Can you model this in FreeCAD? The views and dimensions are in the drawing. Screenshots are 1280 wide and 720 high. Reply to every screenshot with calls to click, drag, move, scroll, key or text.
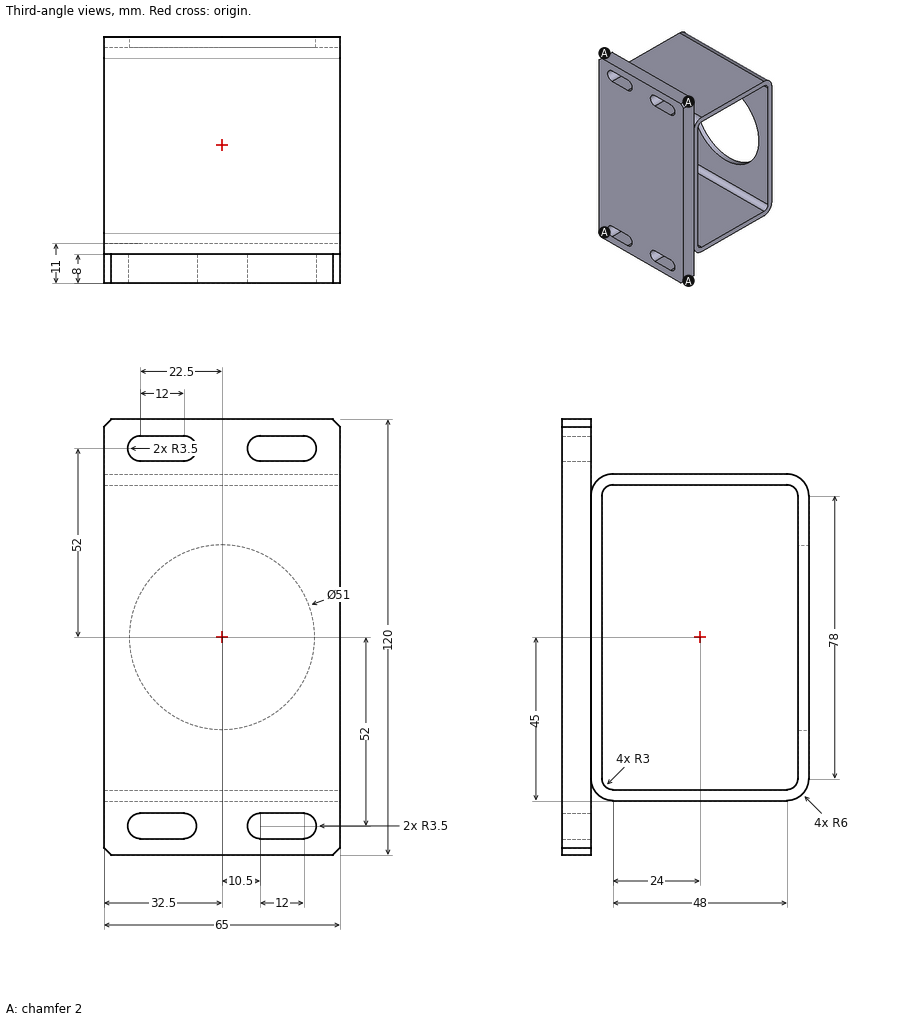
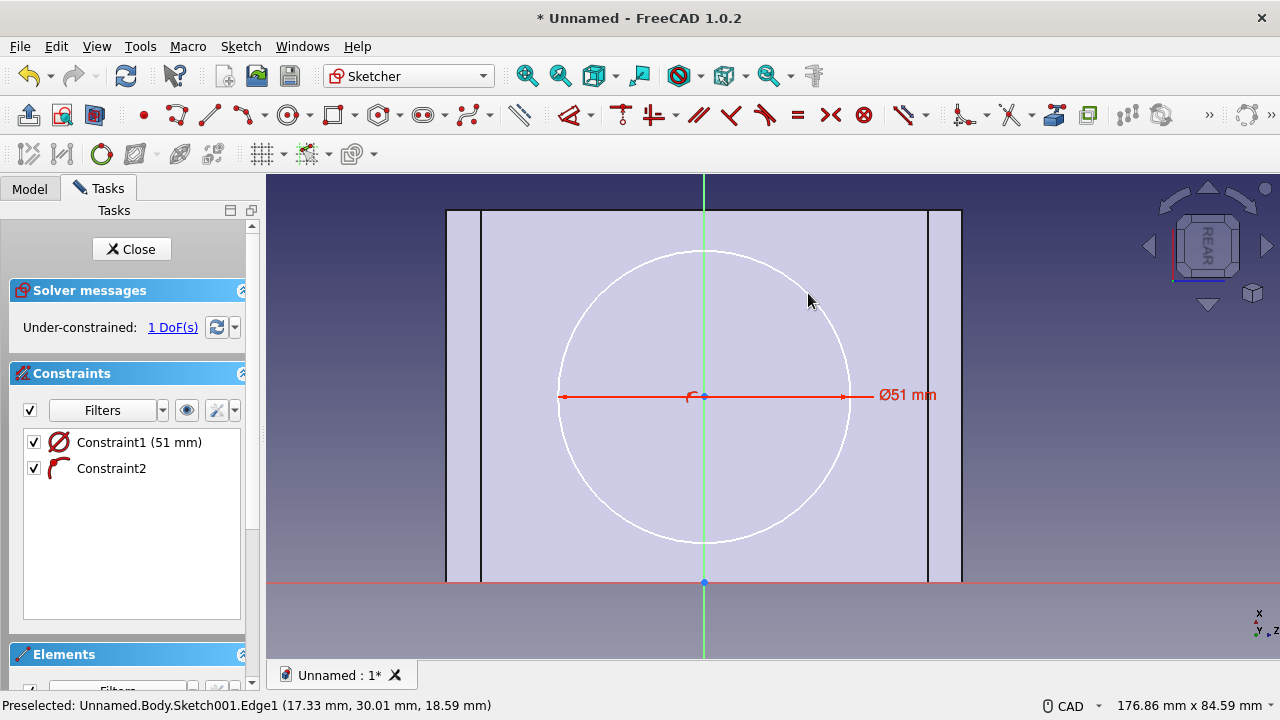
click(568, 116)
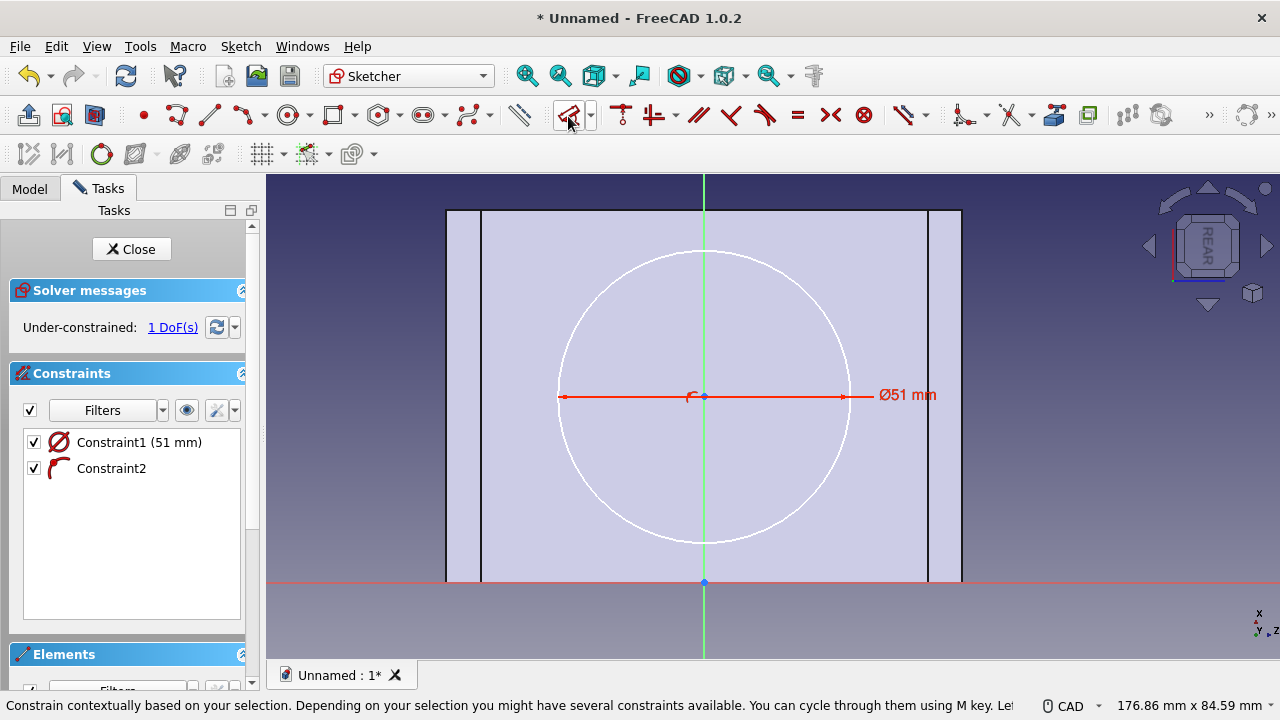
click(704, 397)
click(738, 490)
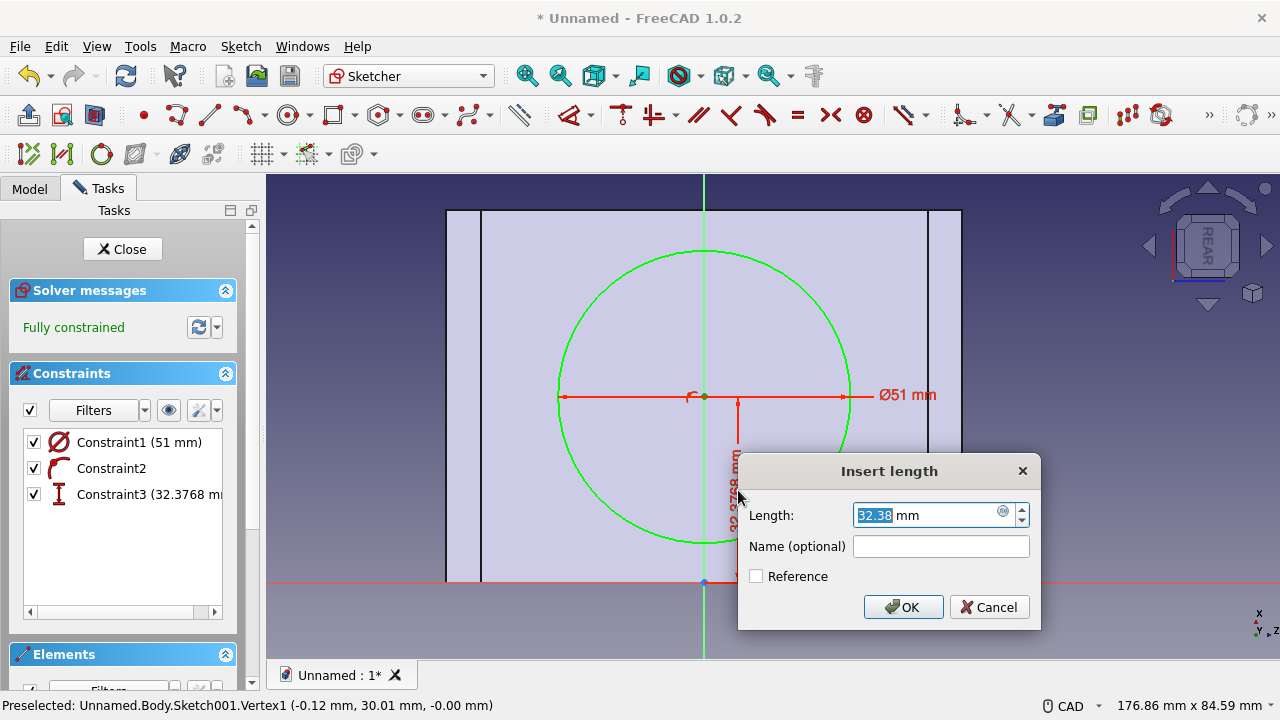
text(32.5)
key(Return)
key(Escape)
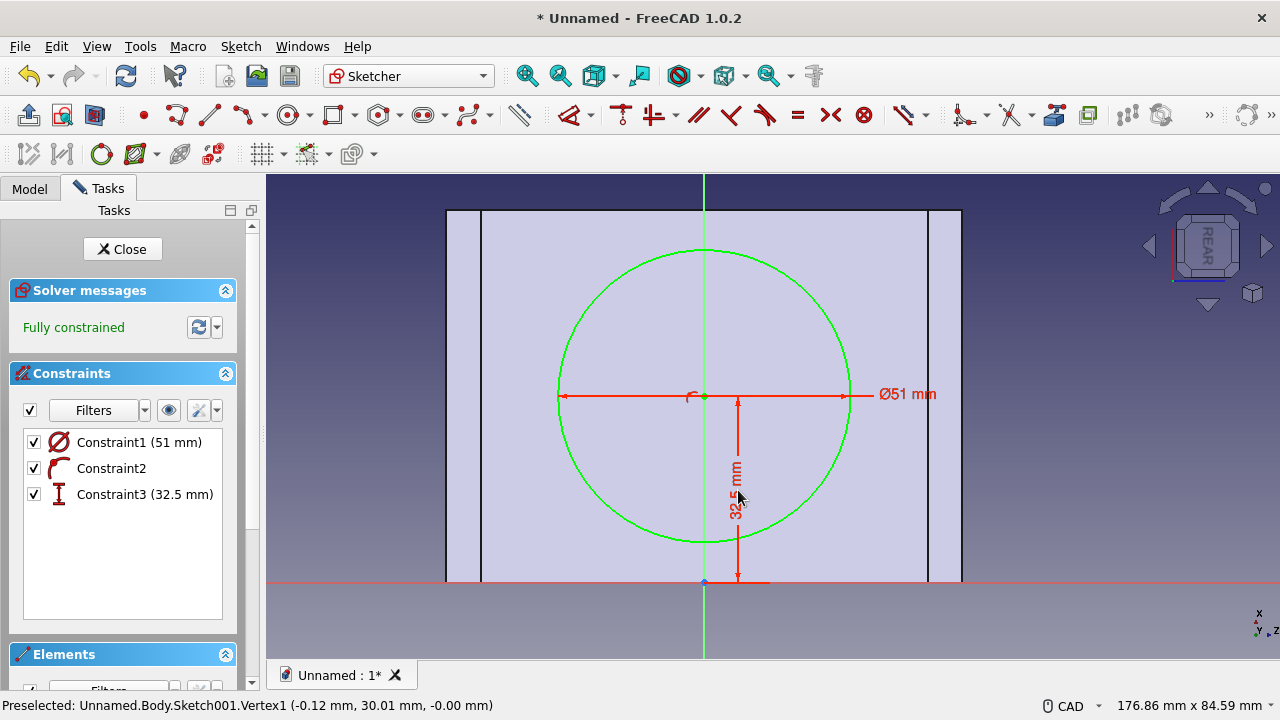
click(123, 249)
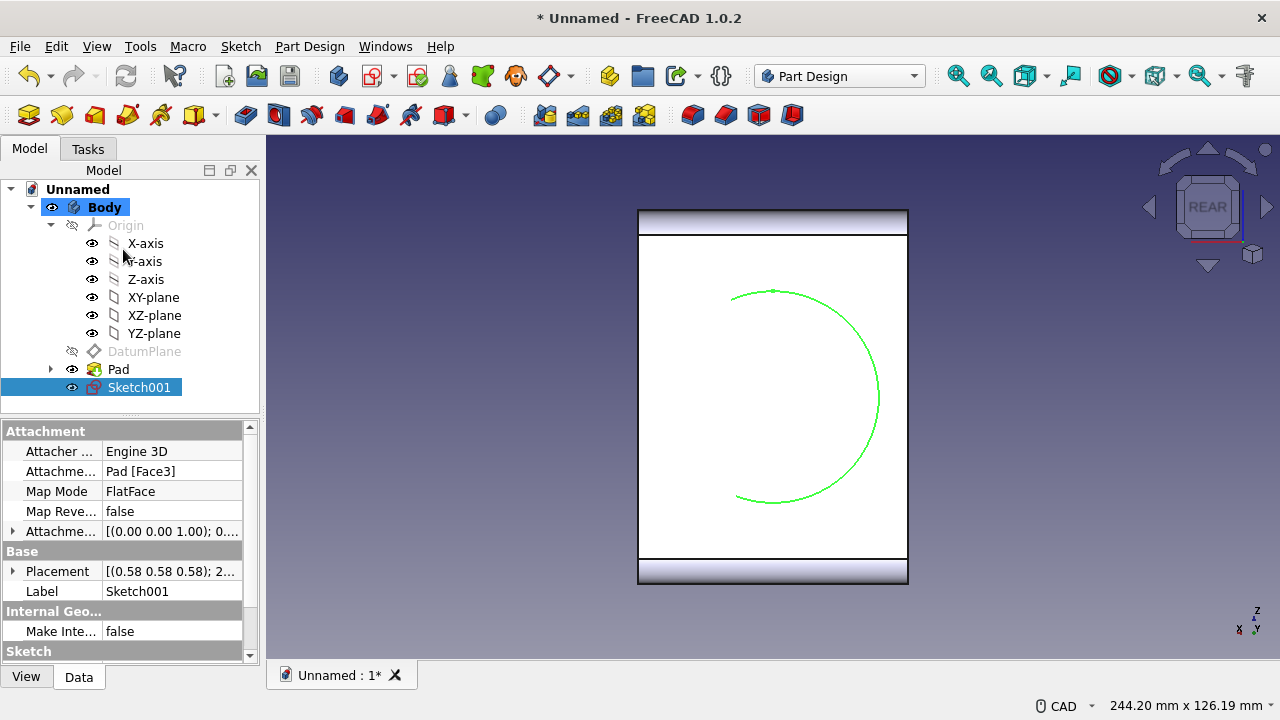
click(246, 116)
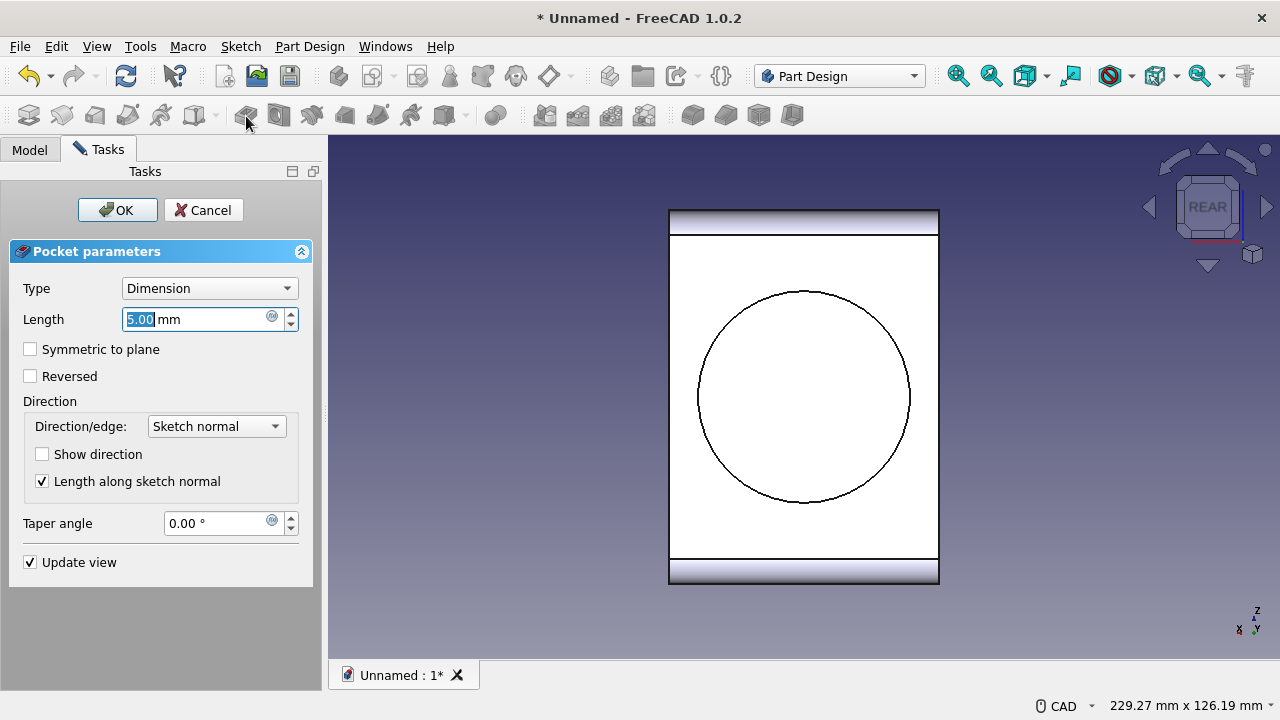
click(210, 288)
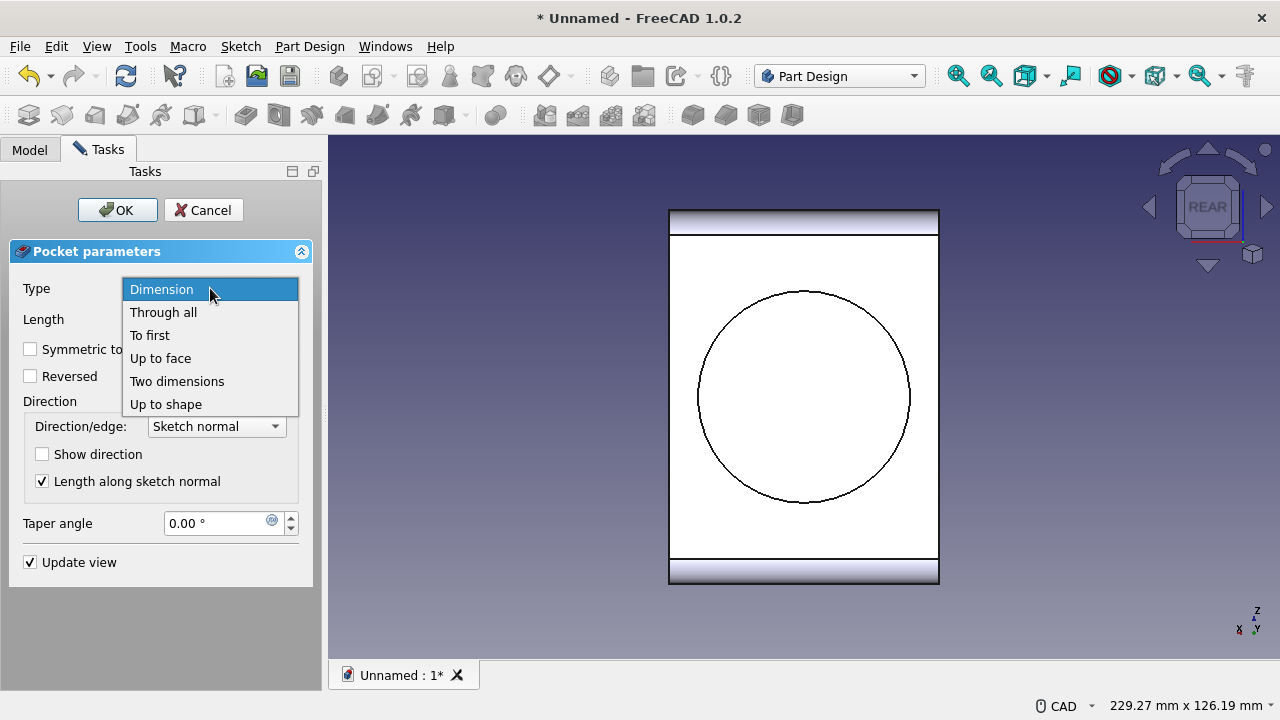
click(208, 336)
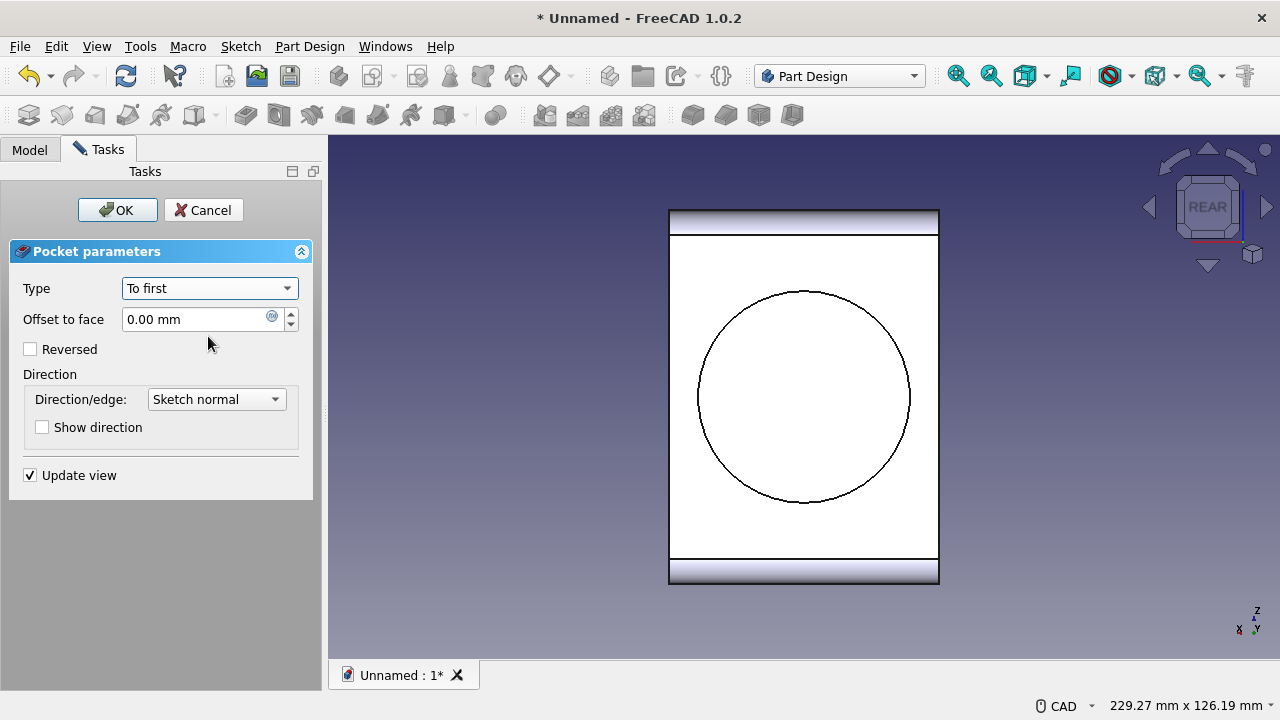
click(118, 210)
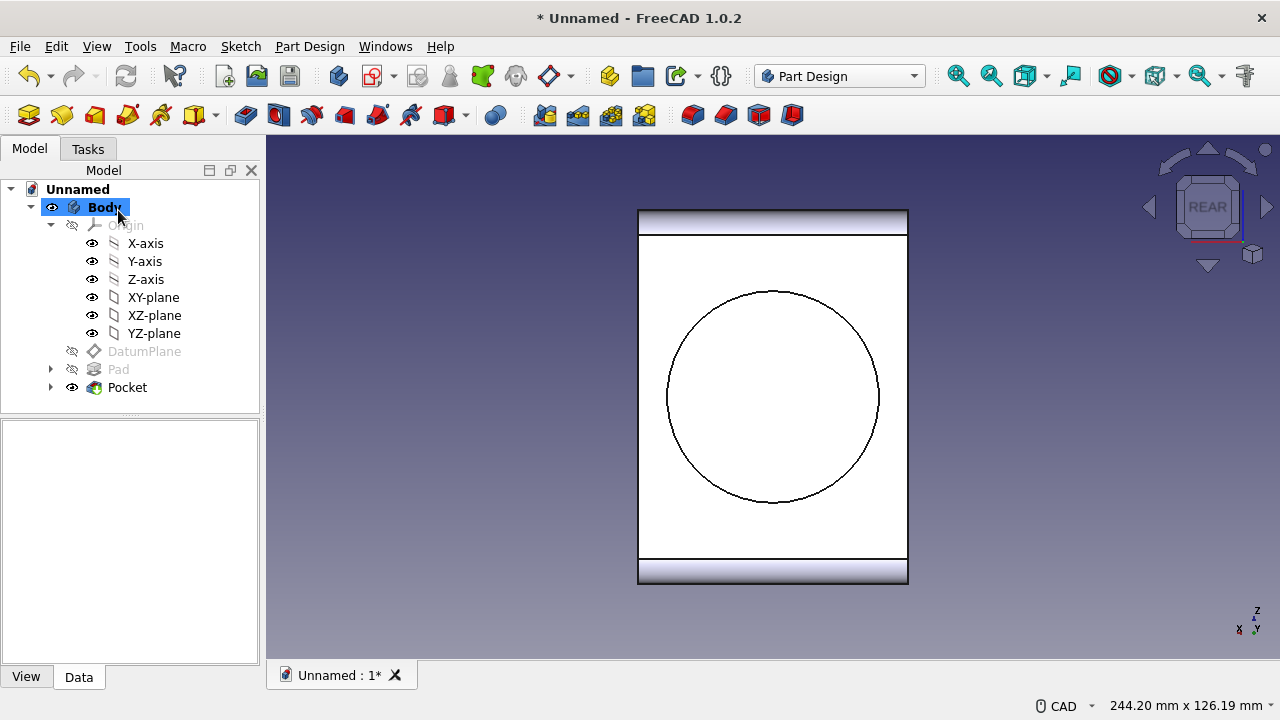
click(339, 76)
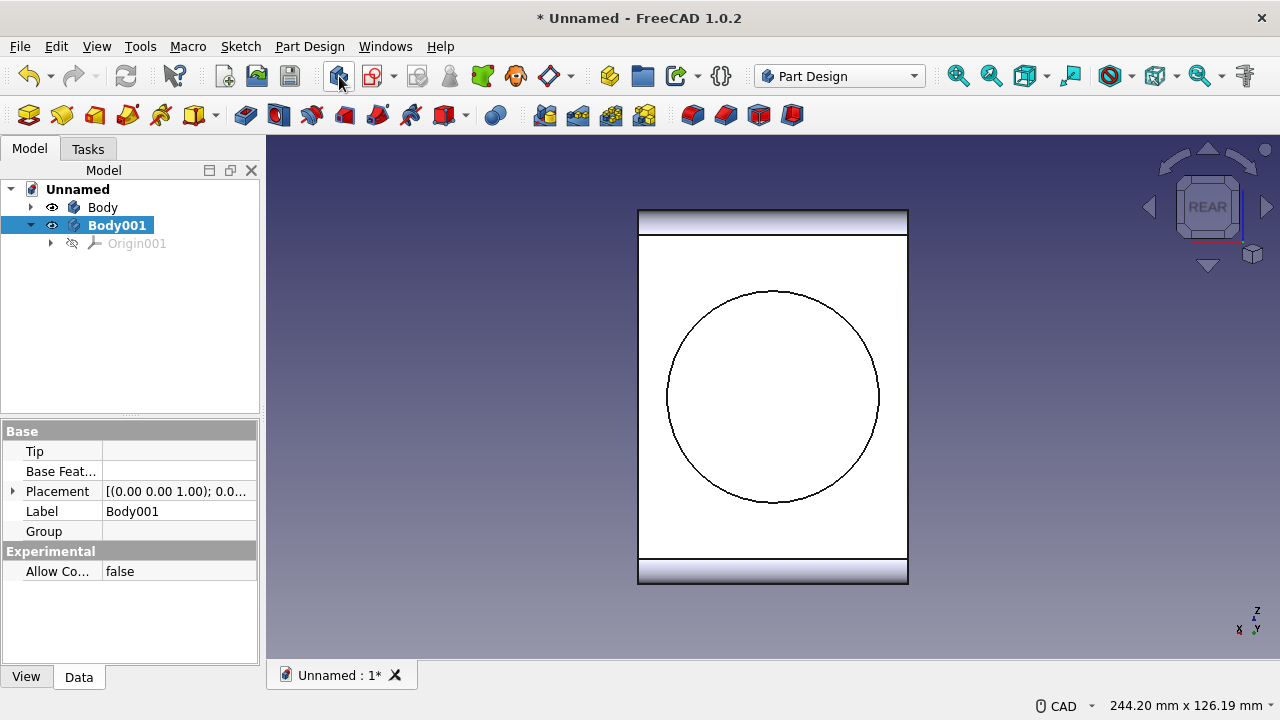
click(51, 243)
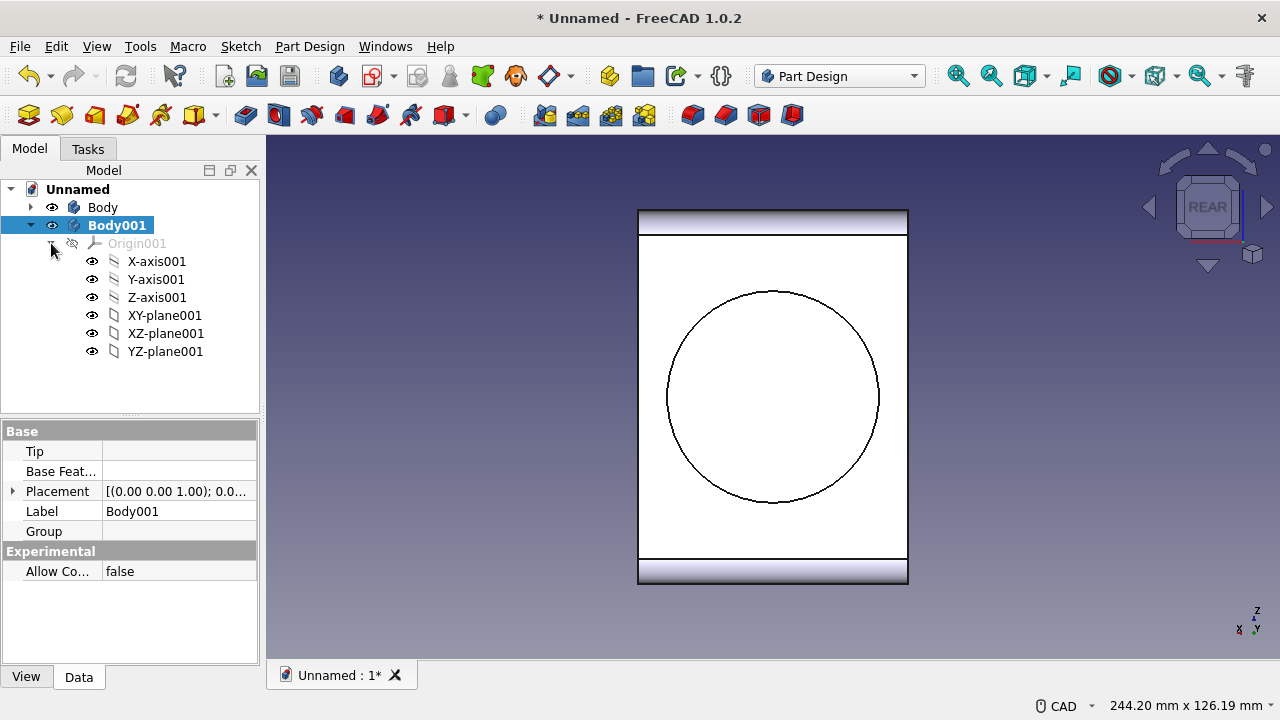
click(137, 333)